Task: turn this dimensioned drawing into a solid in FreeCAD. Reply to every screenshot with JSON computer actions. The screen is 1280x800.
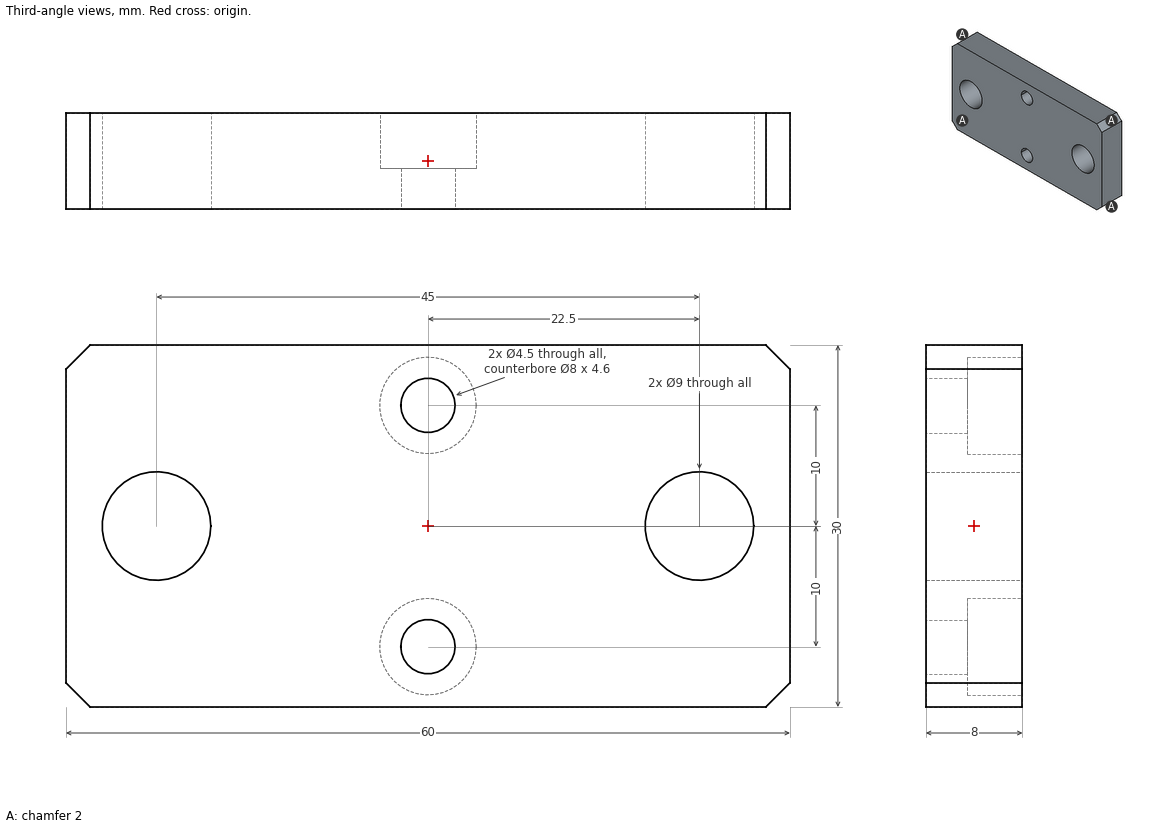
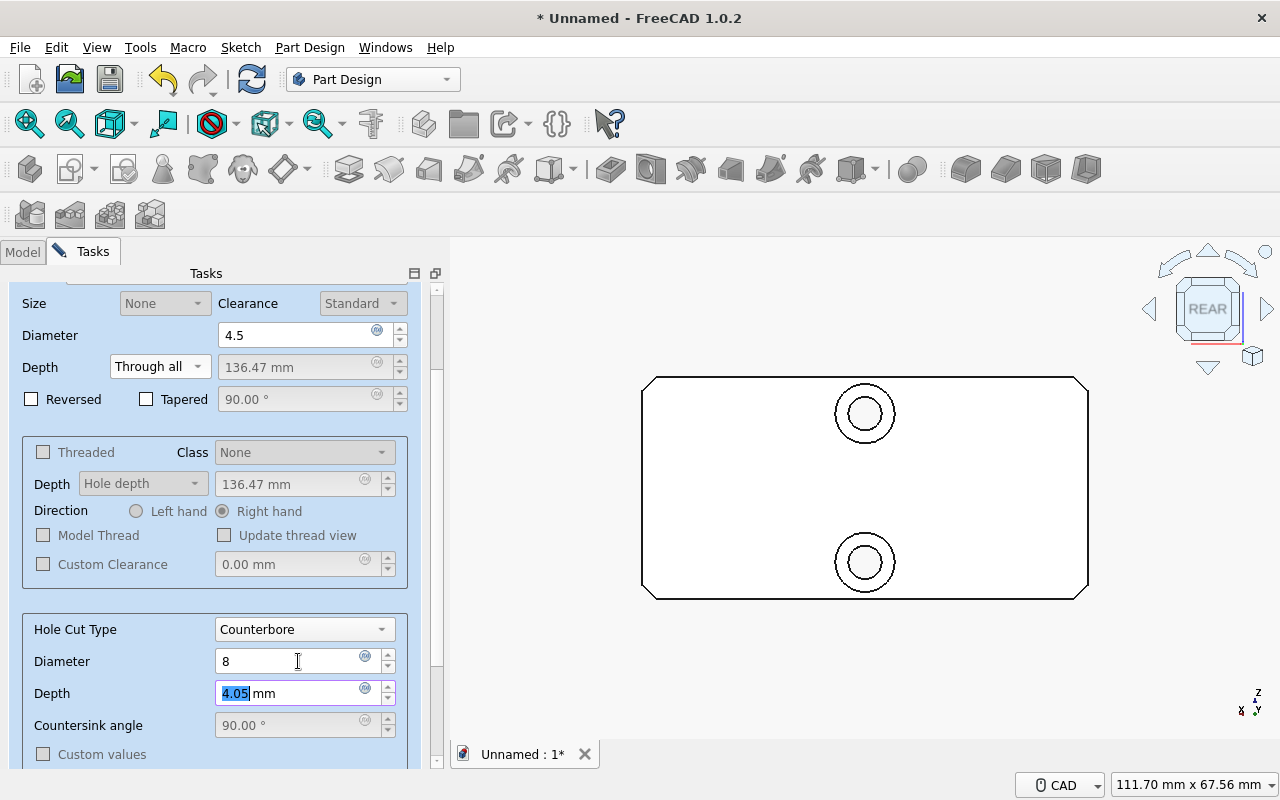
{"action": "type", "text": "4.6"}
{"action": "key", "text": "Tab"}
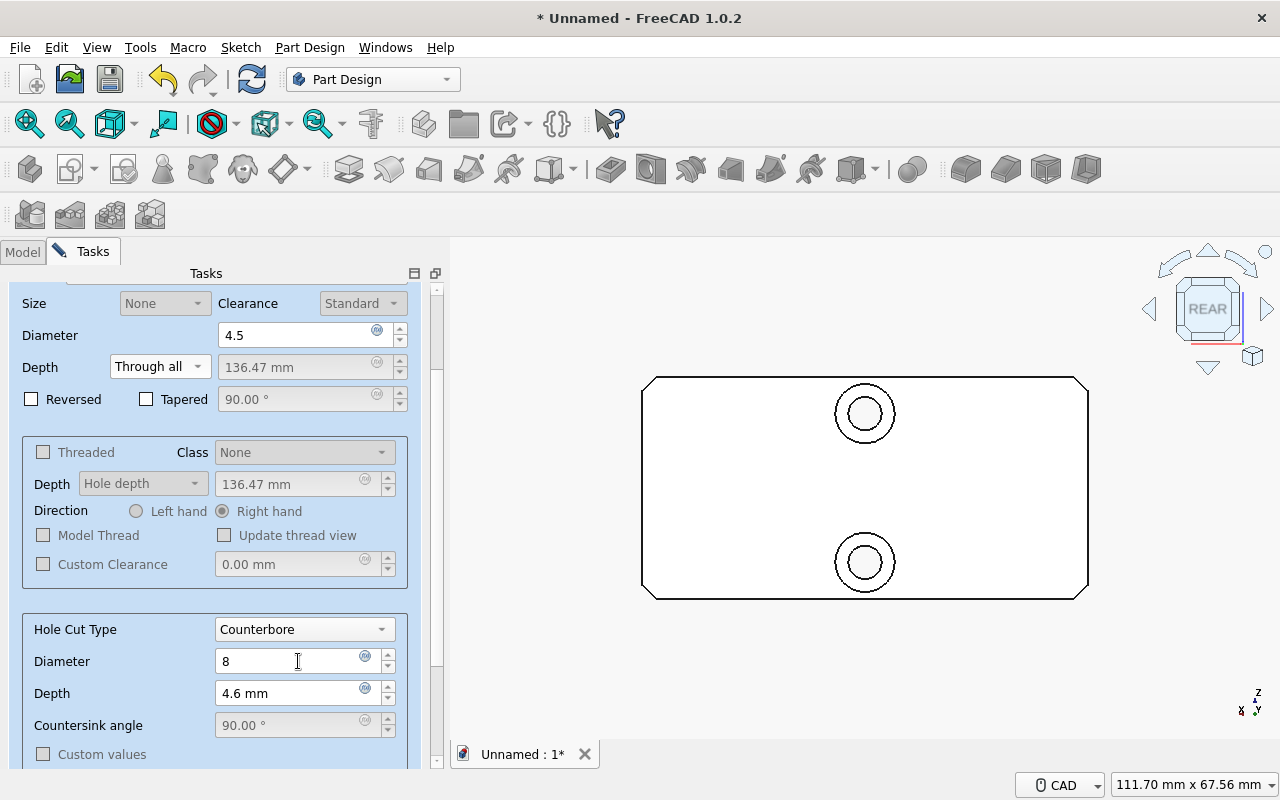
{"action": "scroll", "coordinate": [437, 526], "scroll_direction": "up", "scroll_amount": 3}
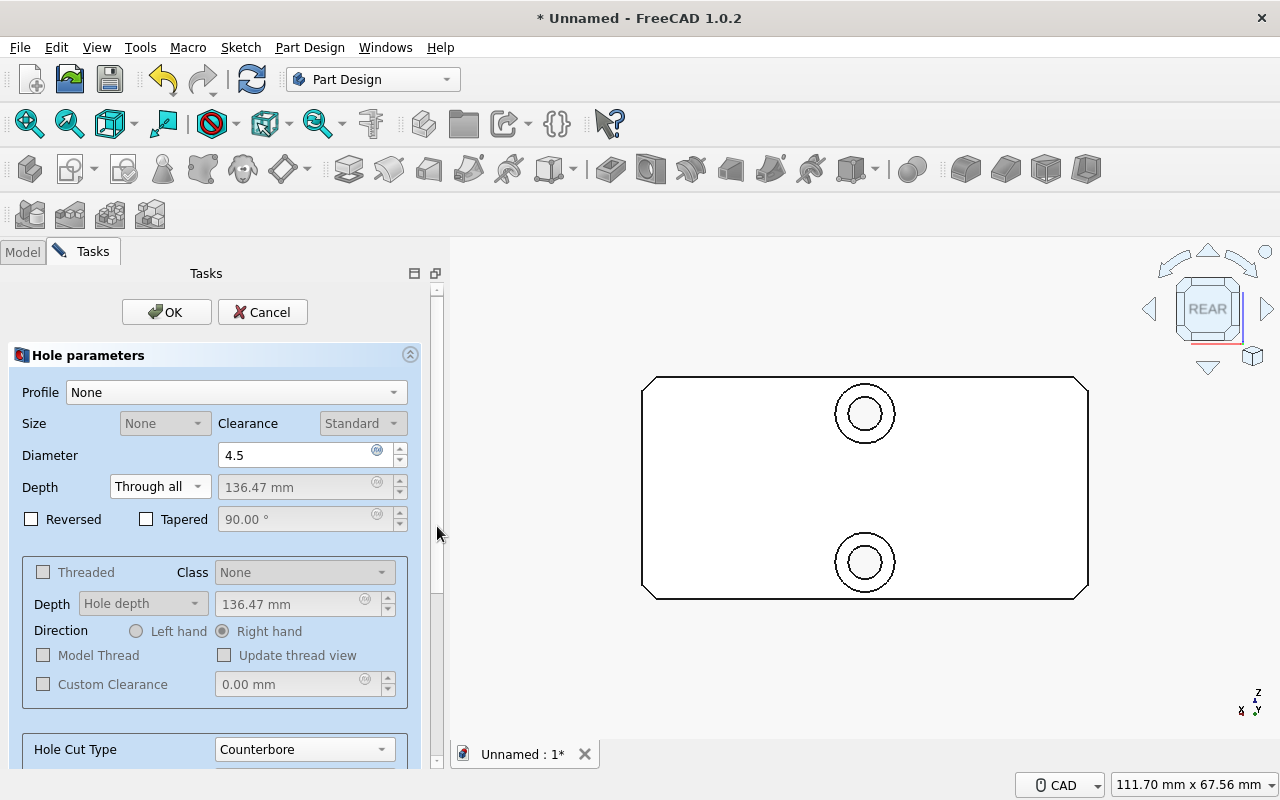
{"action": "left_click", "coordinate": [167, 312]}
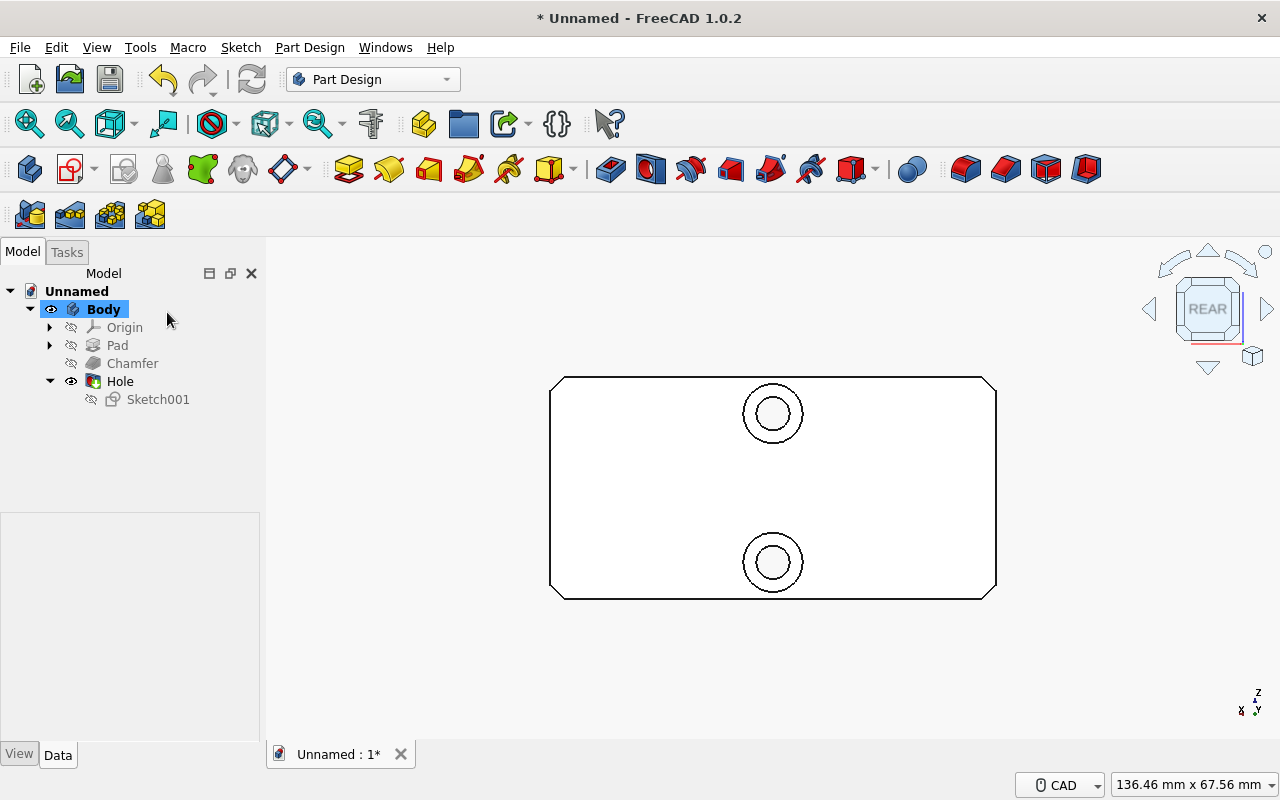
{"action": "left_click", "coordinate": [30, 124]}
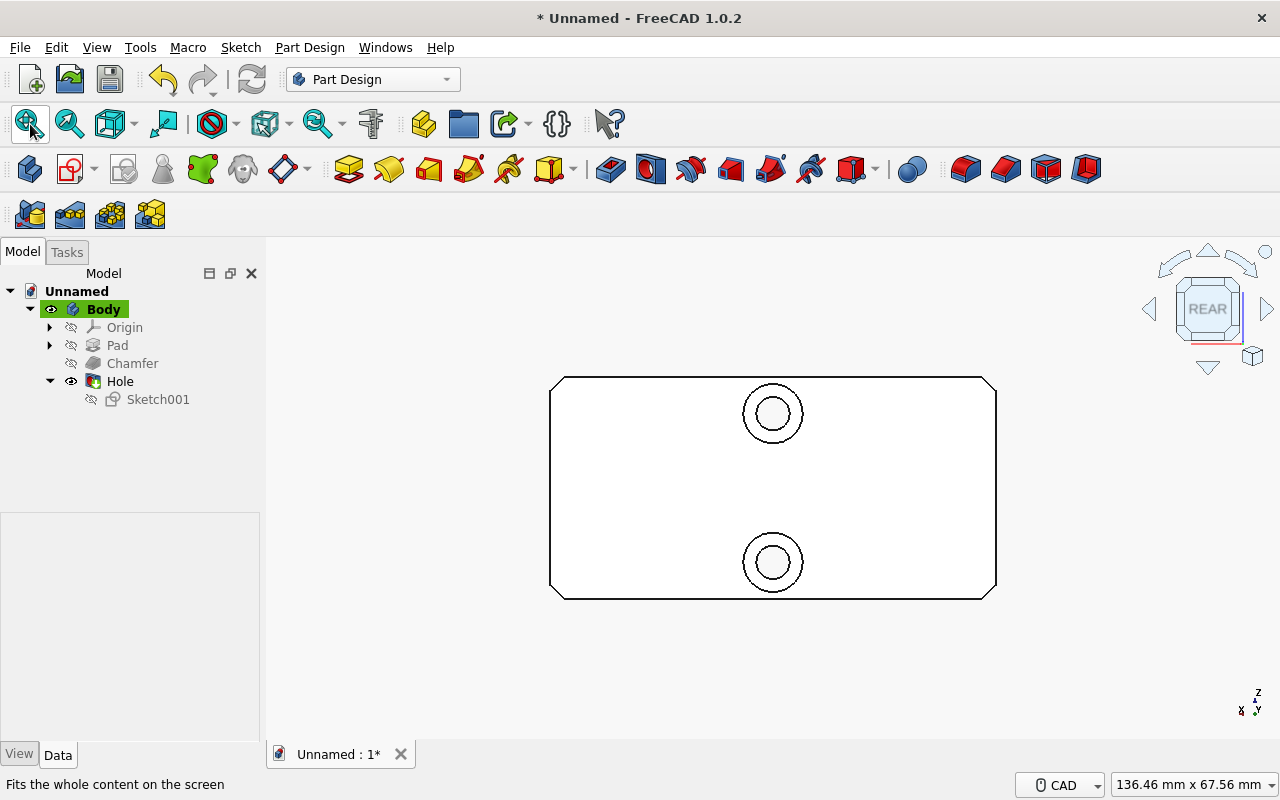
{"action": "key", "text": "0"}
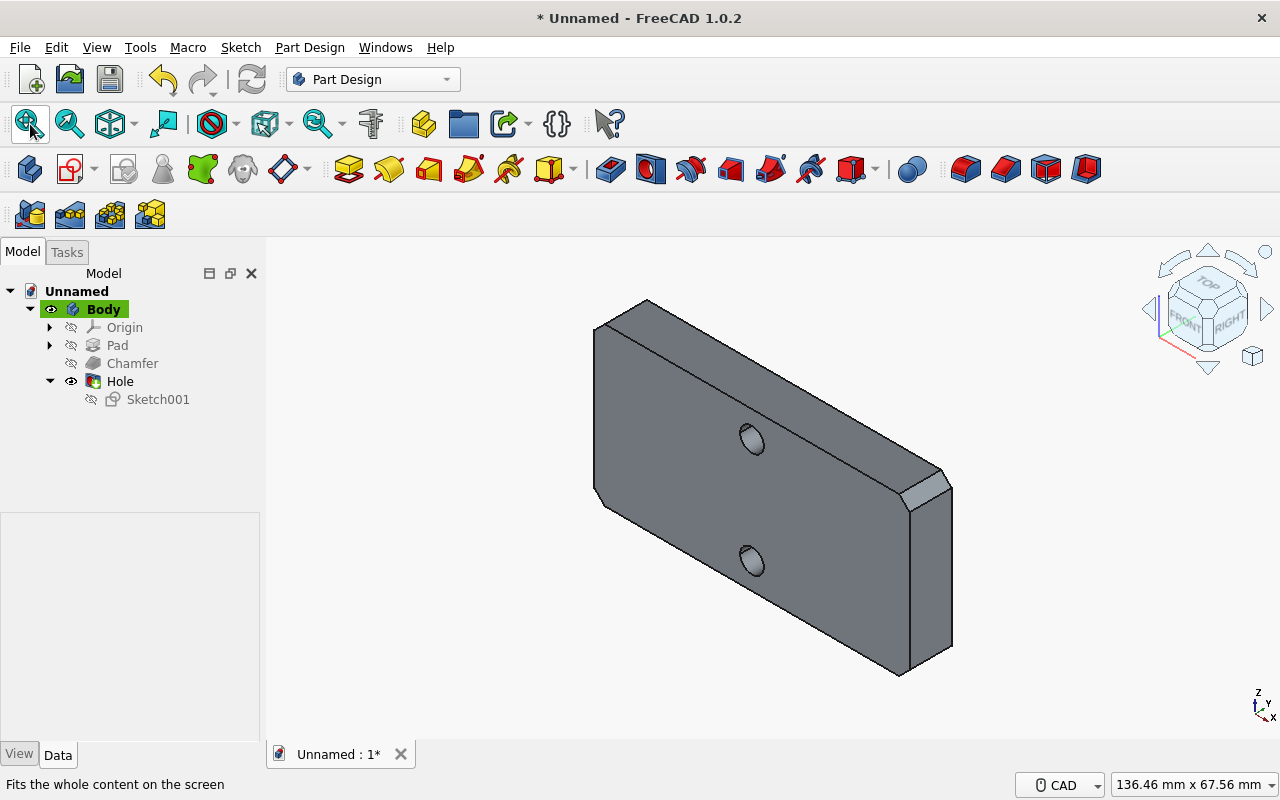
{"action": "left_click", "coordinate": [662, 447]}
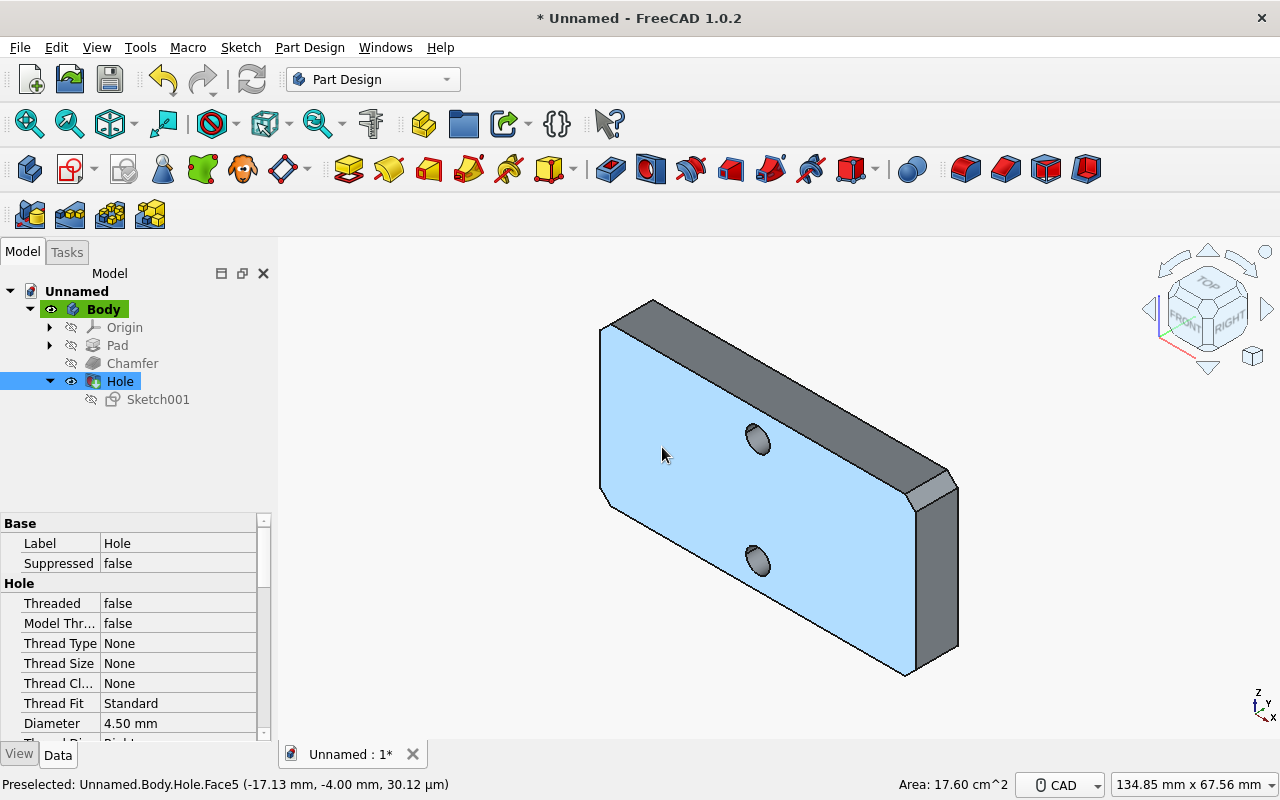
{"action": "left_click", "coordinate": [70, 170]}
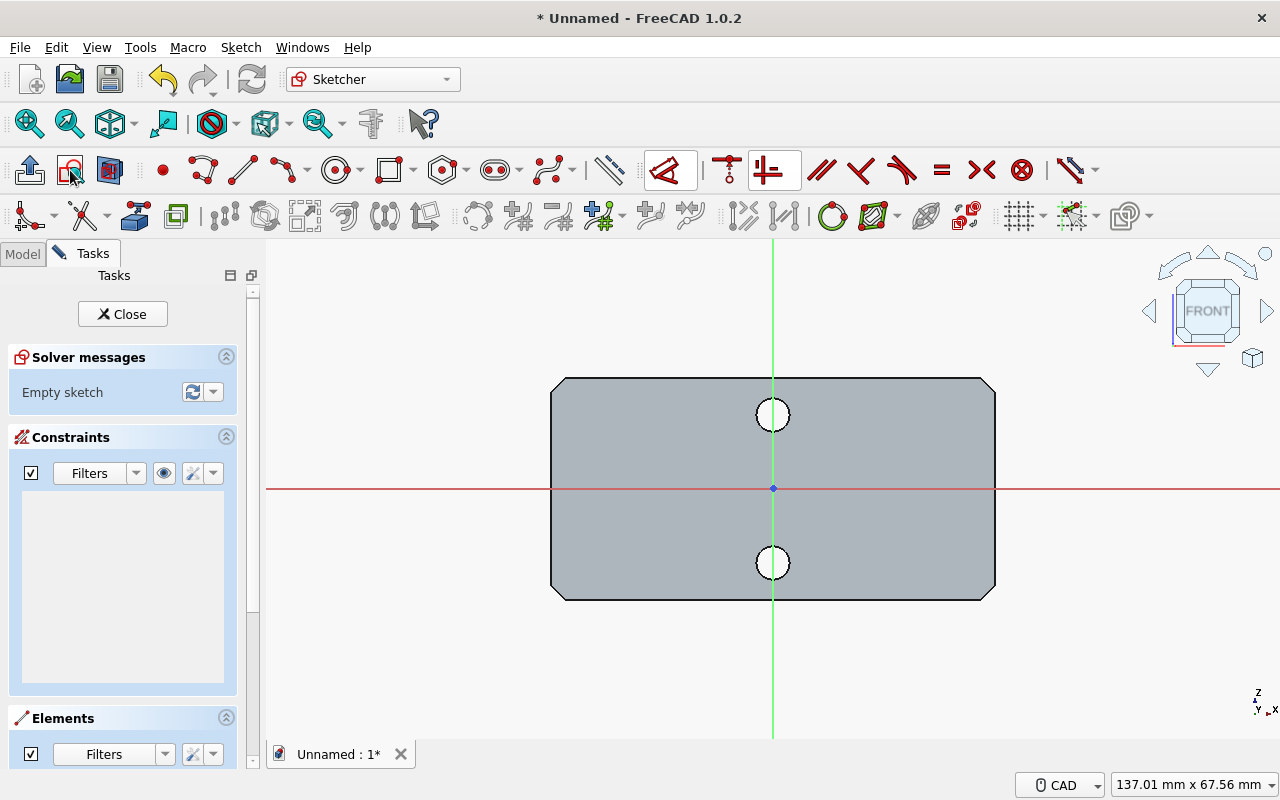
{"action": "scroll", "coordinate": [912, 489], "scroll_direction": "up", "scroll_amount": 2}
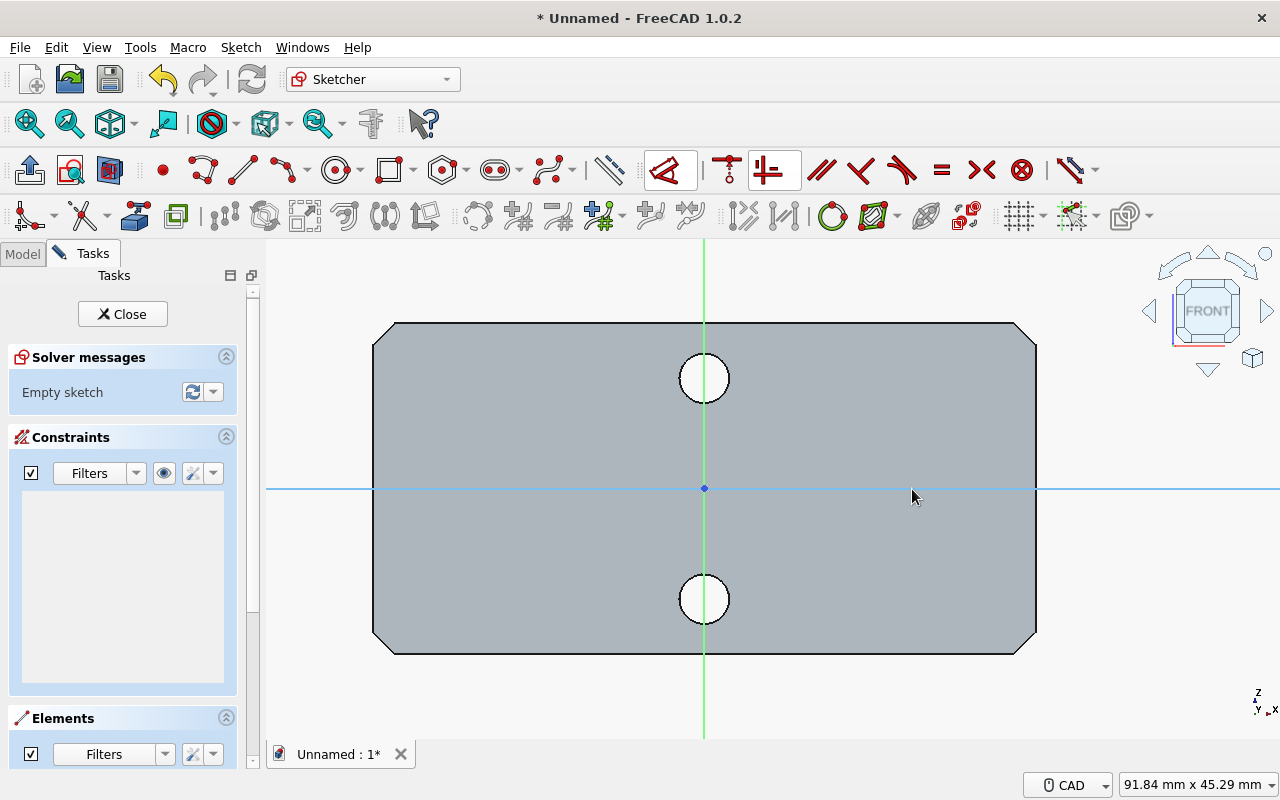
{"action": "left_click", "coordinate": [336, 170]}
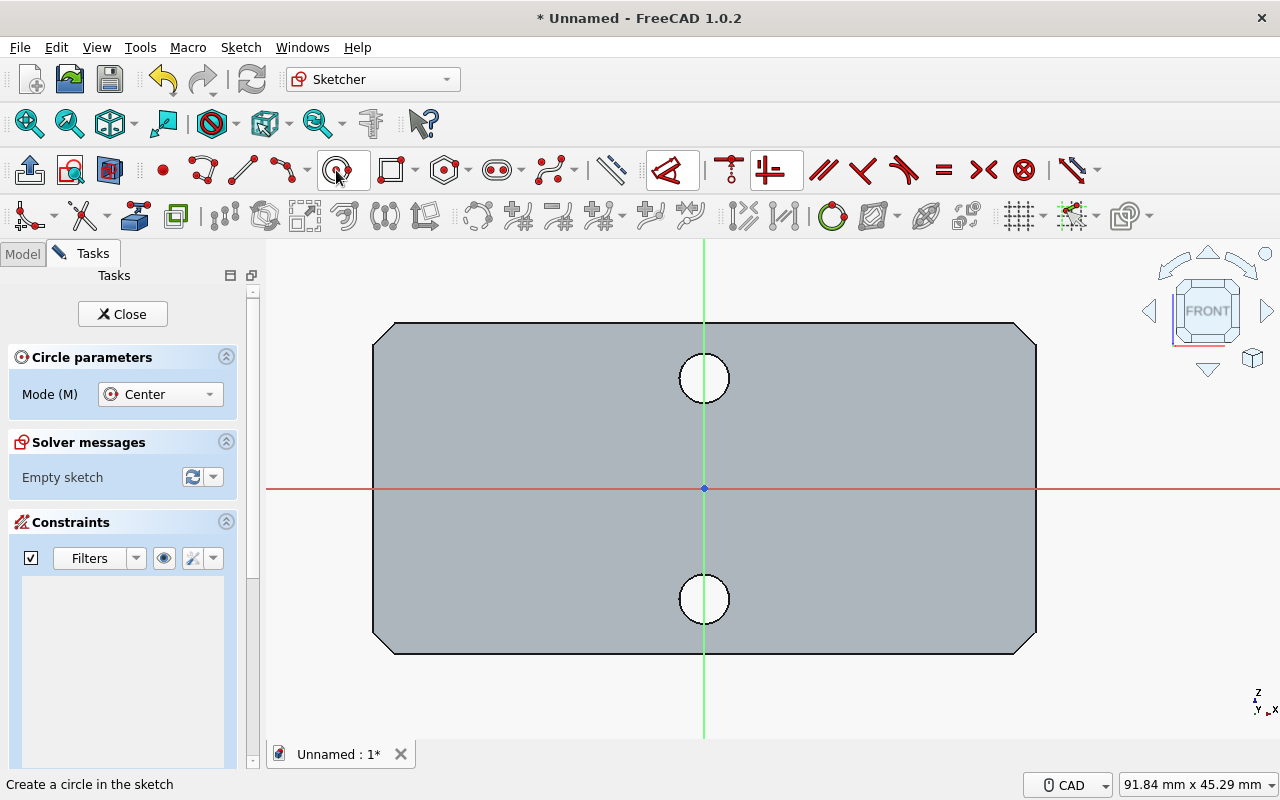
{"action": "left_click", "coordinate": [953, 489]}
{"action": "left_click", "coordinate": [988, 454]}